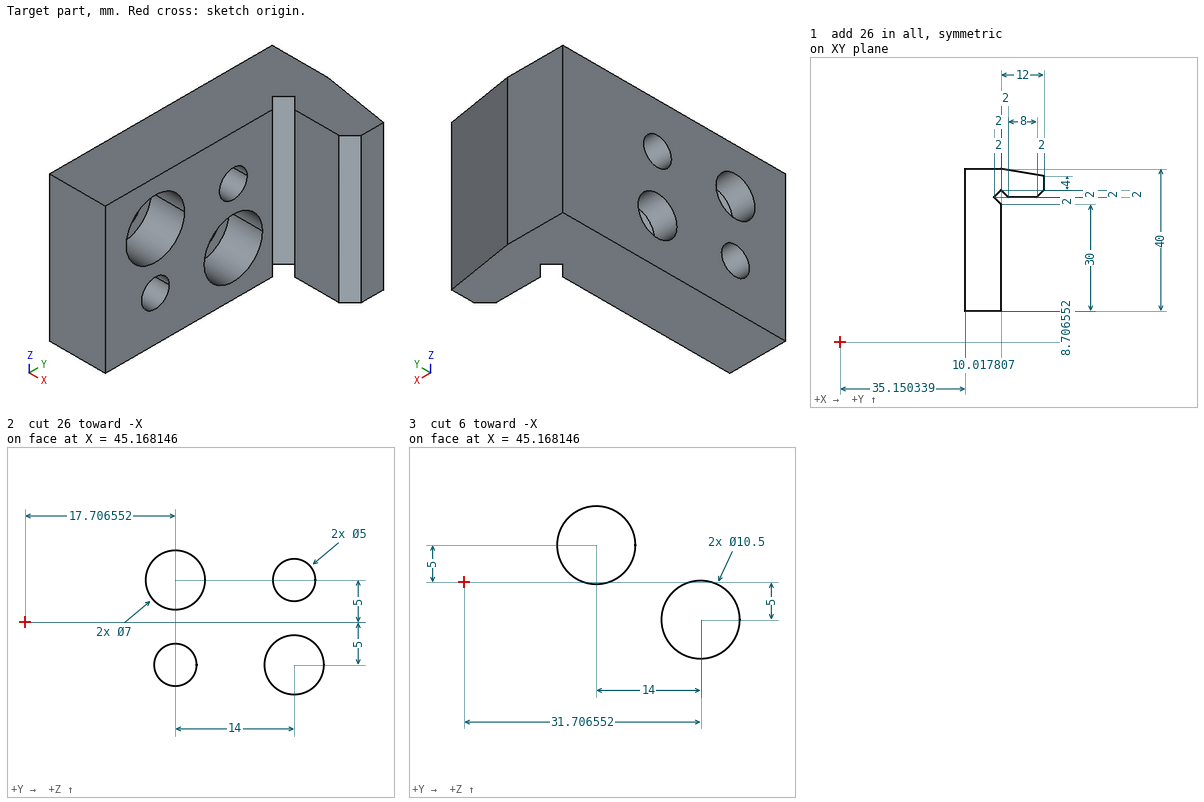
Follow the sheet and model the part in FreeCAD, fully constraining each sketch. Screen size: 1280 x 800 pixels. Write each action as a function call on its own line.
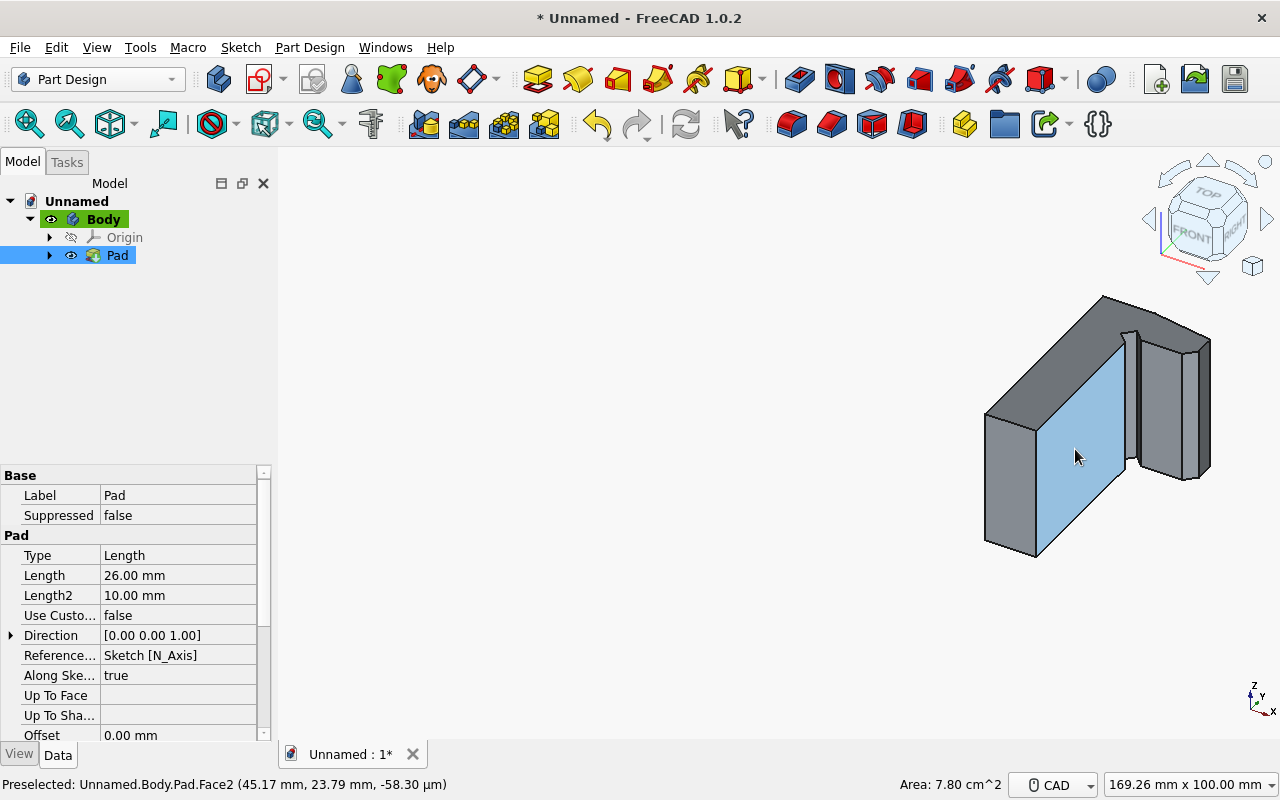
click(260, 80)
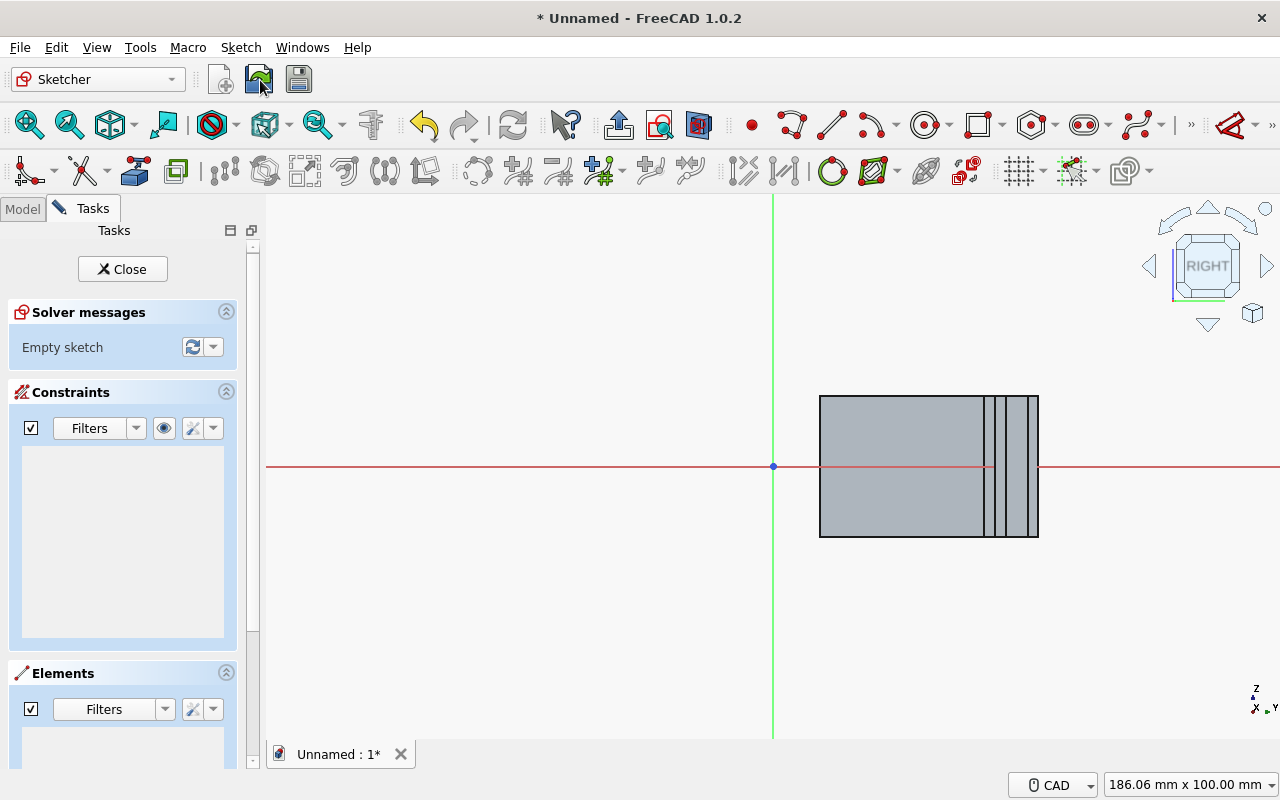
scroll(940, 466, up, 6)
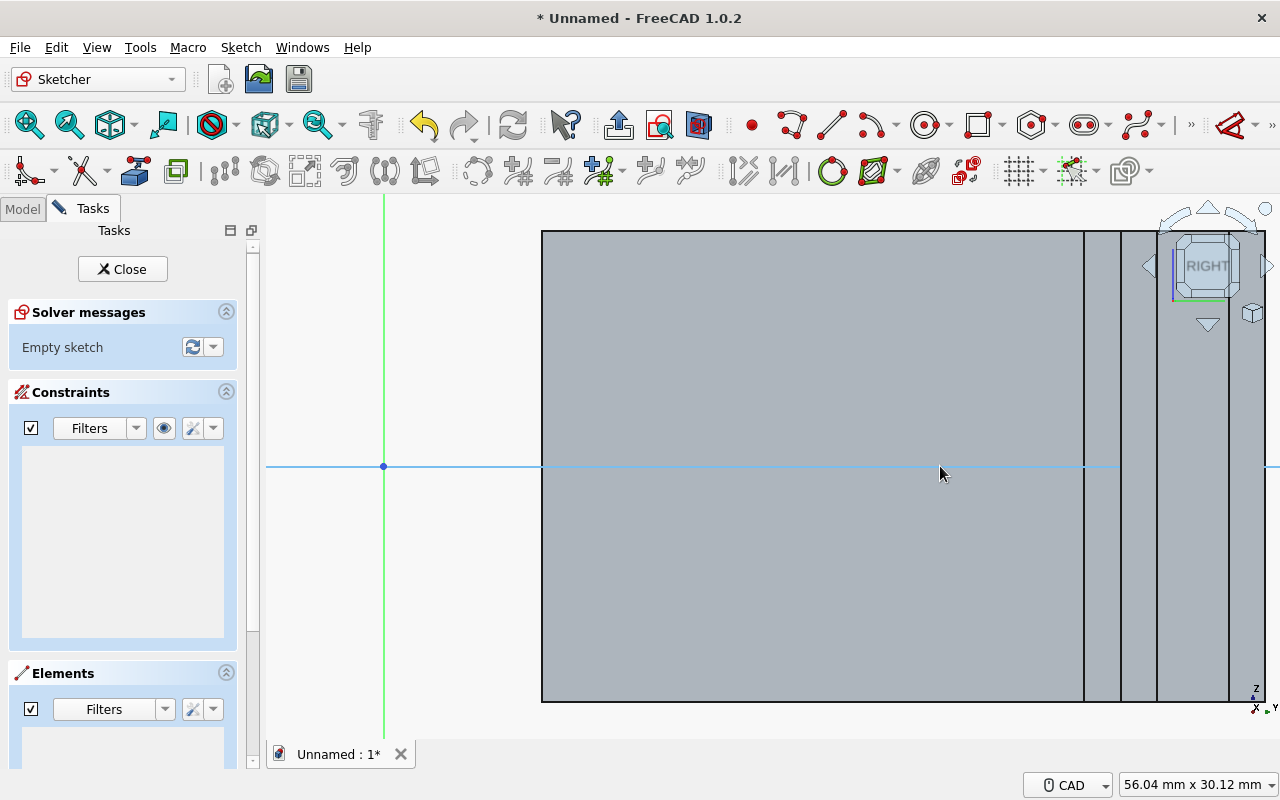
key(g)
key(c)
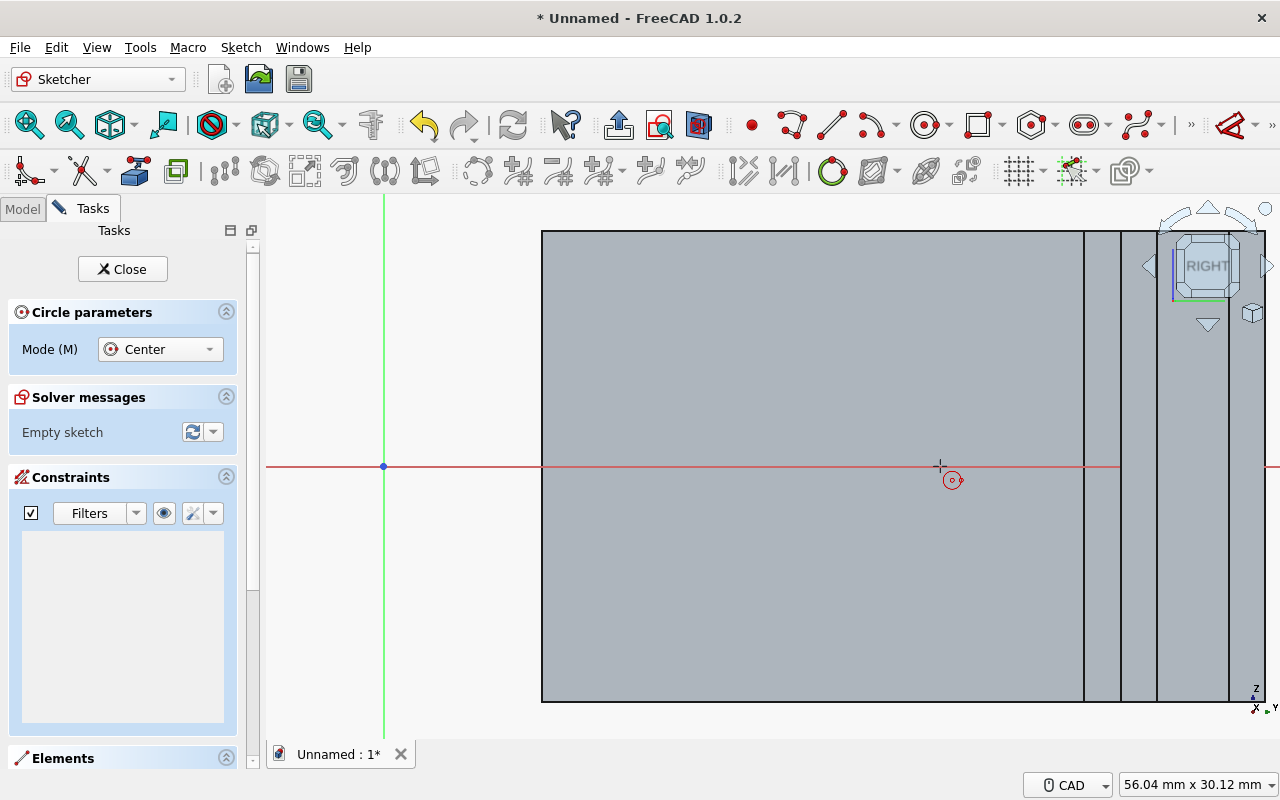
click(704, 376)
move(749, 331)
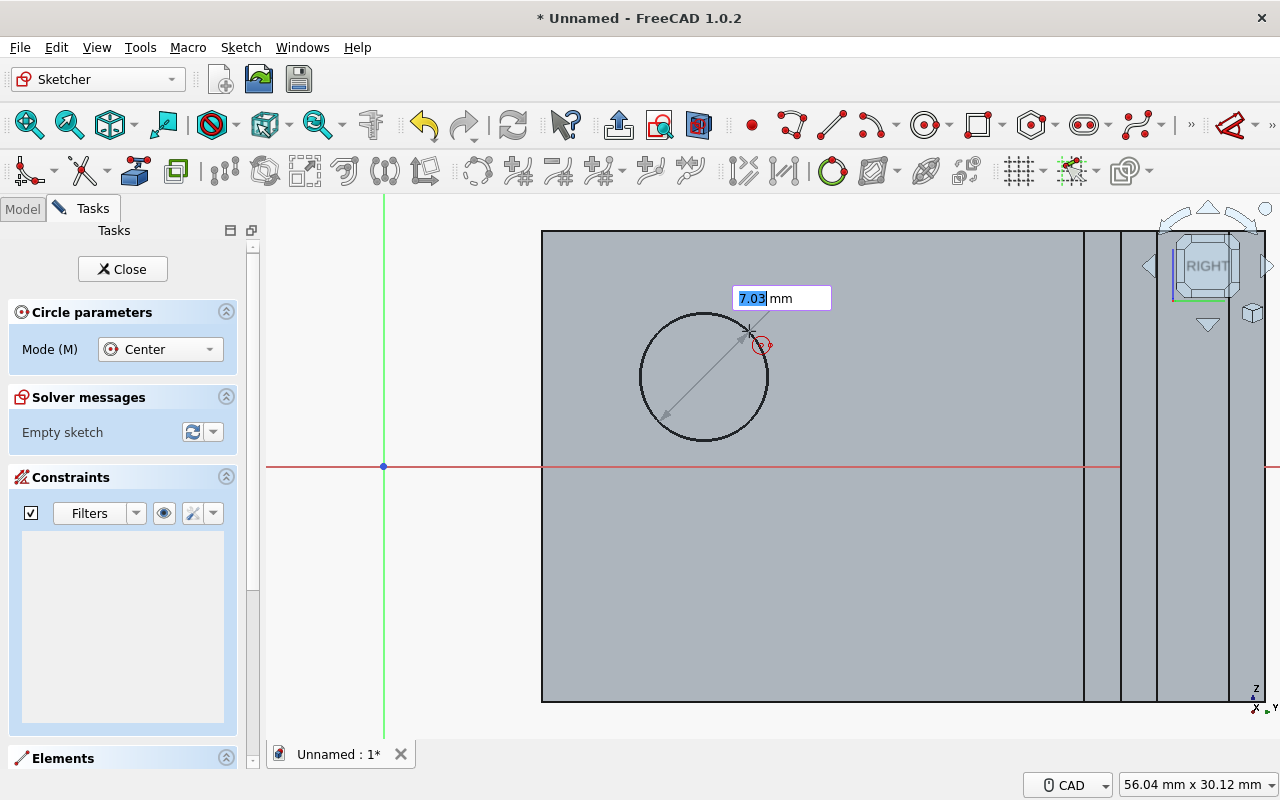
text(7)
key(Return)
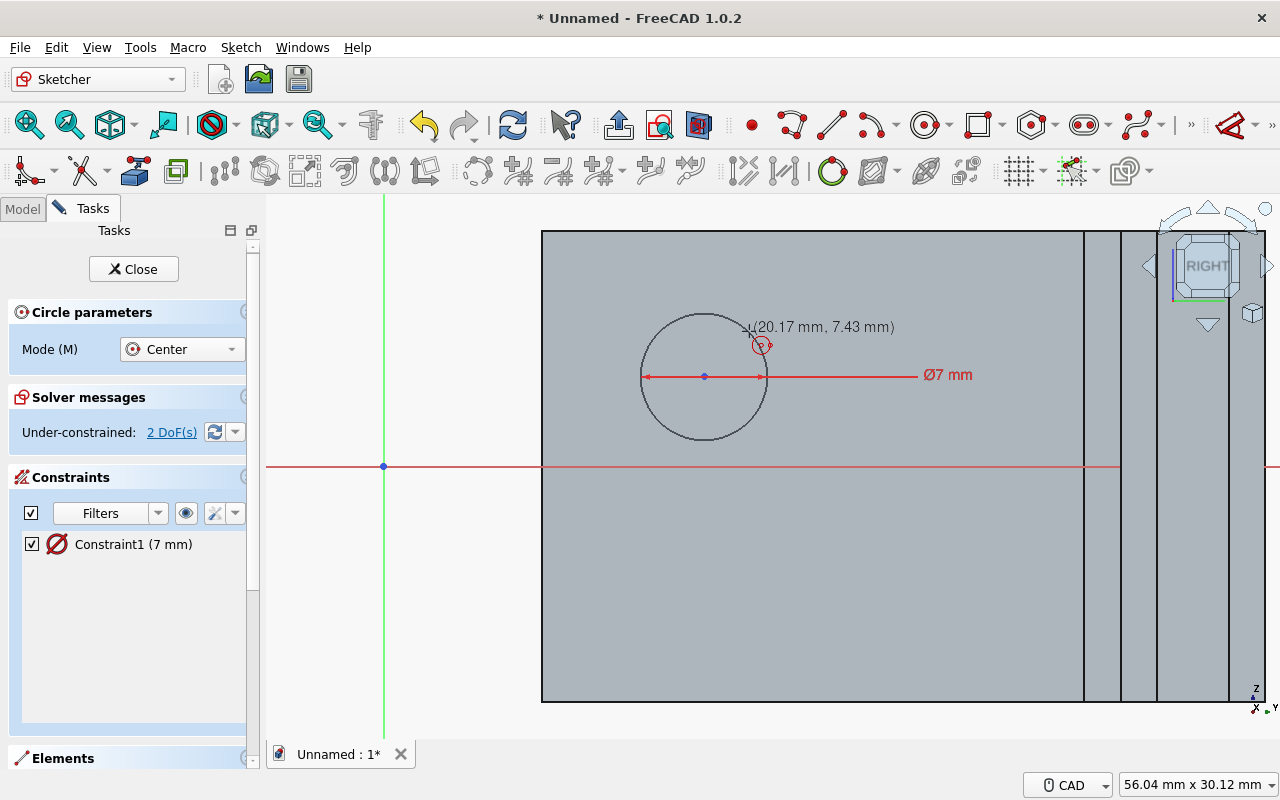
click(958, 557)
move(1002, 512)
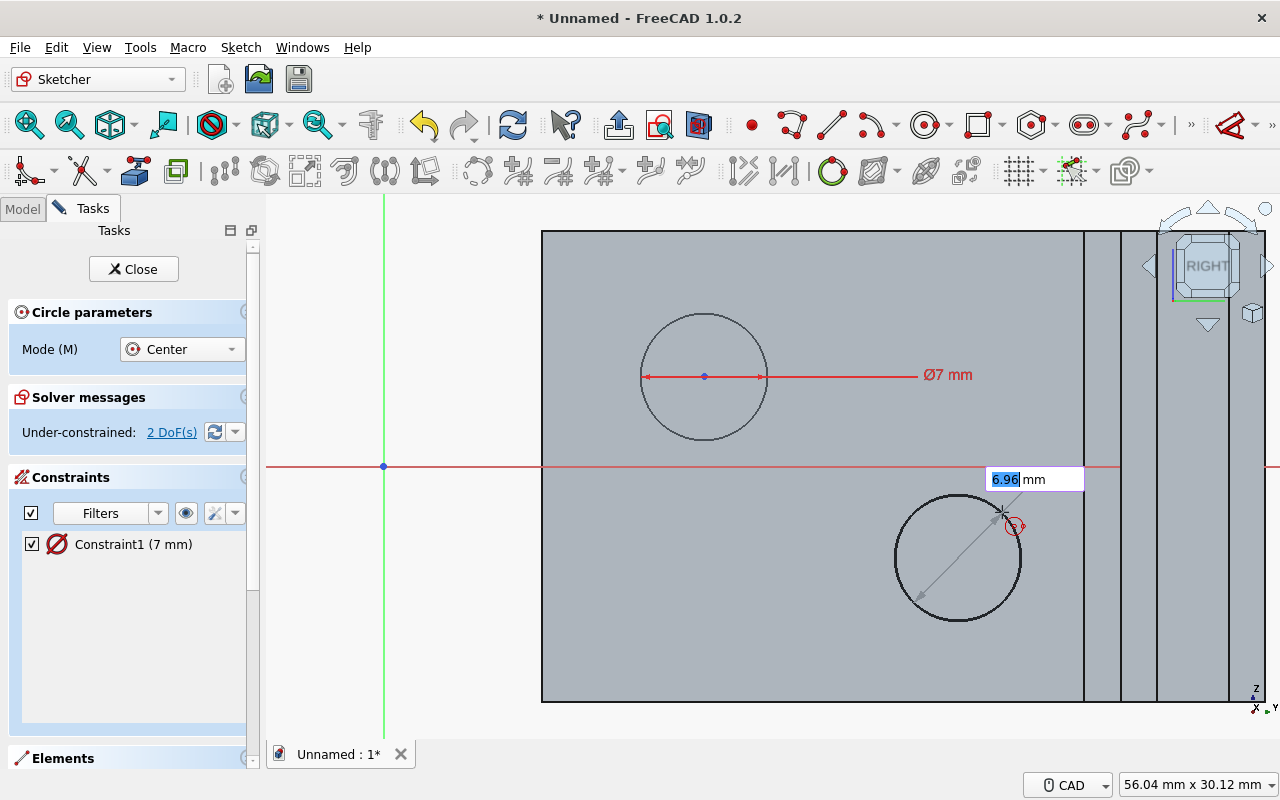
text(7)
key(Return)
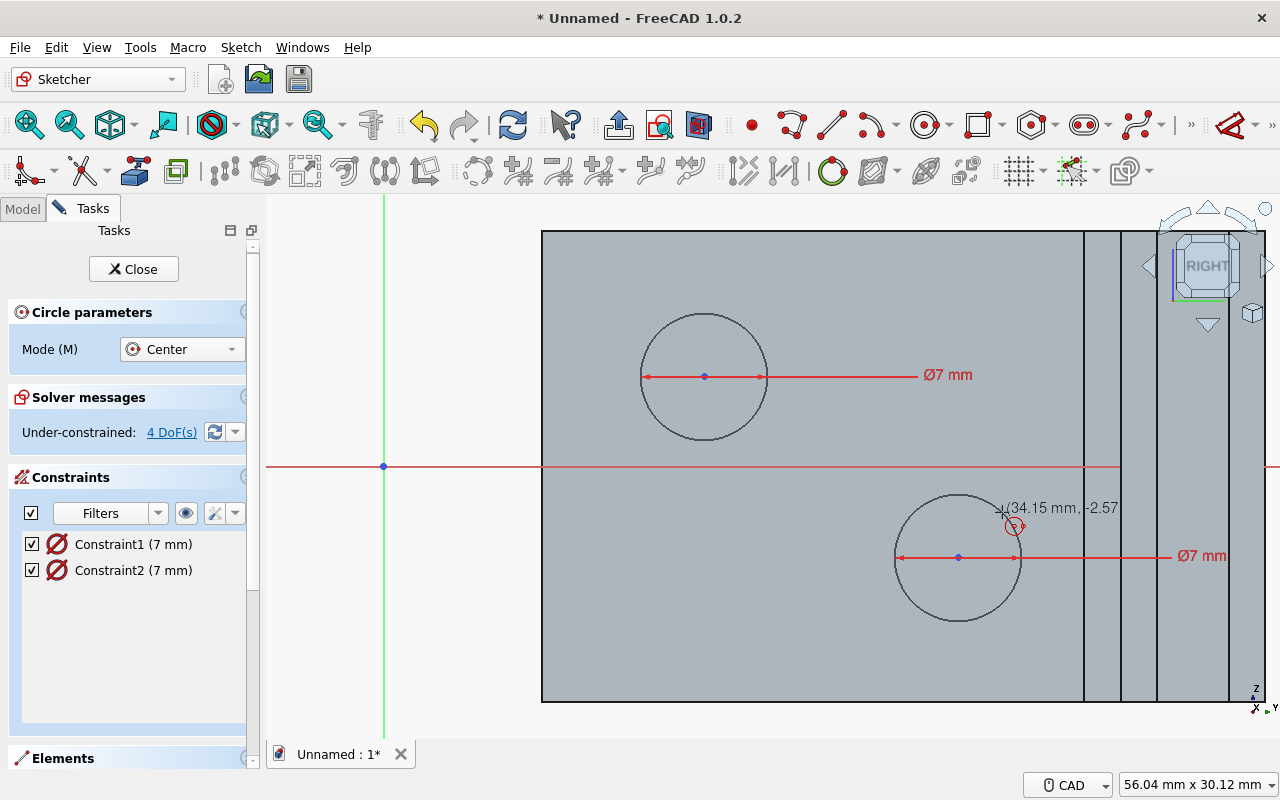
click(704, 557)
move(736, 525)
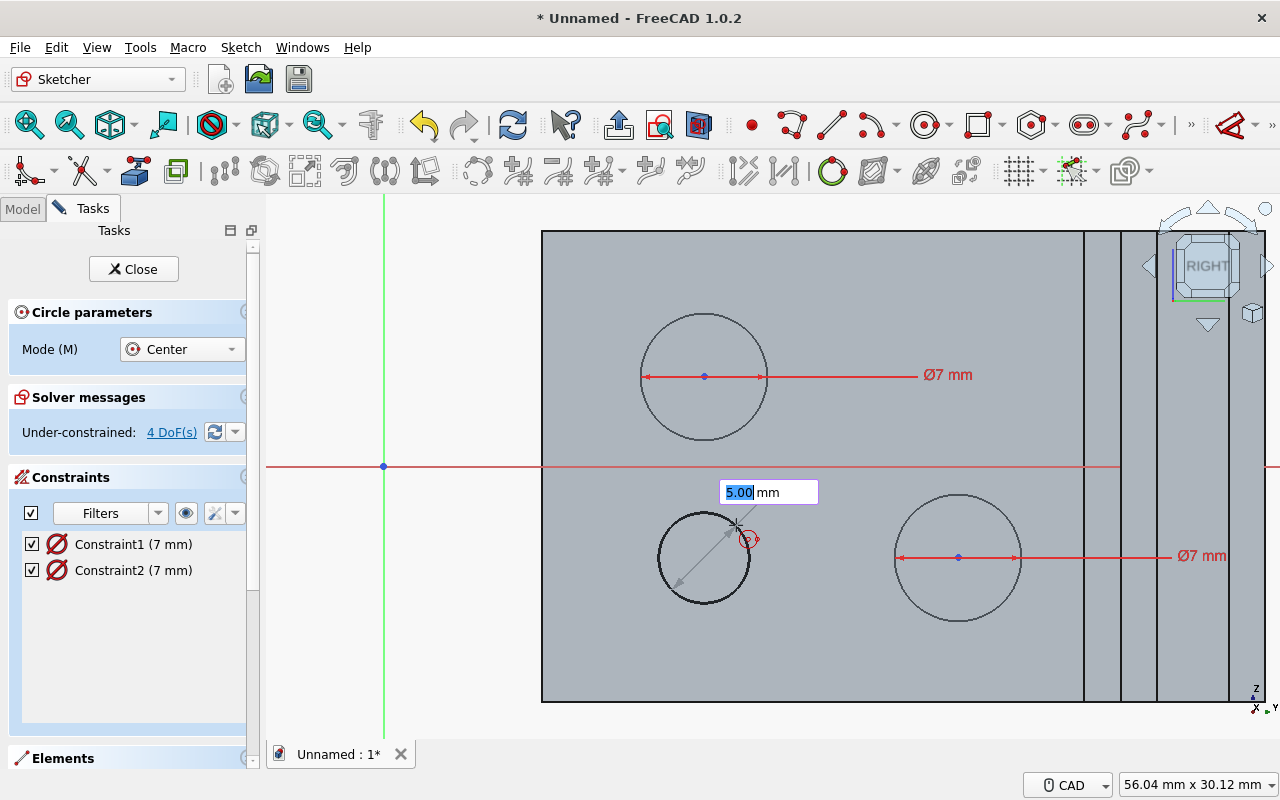
text(5)
key(Return)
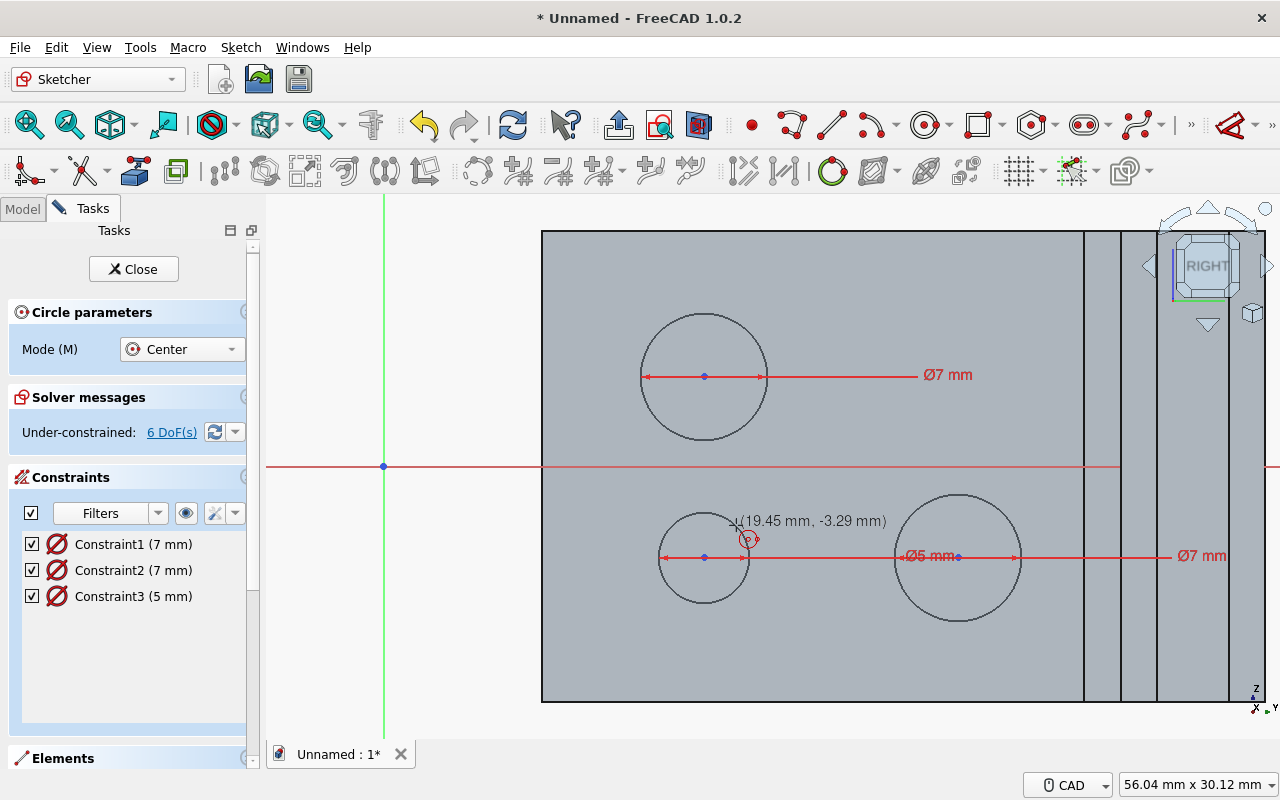
click(958, 376)
move(990, 344)